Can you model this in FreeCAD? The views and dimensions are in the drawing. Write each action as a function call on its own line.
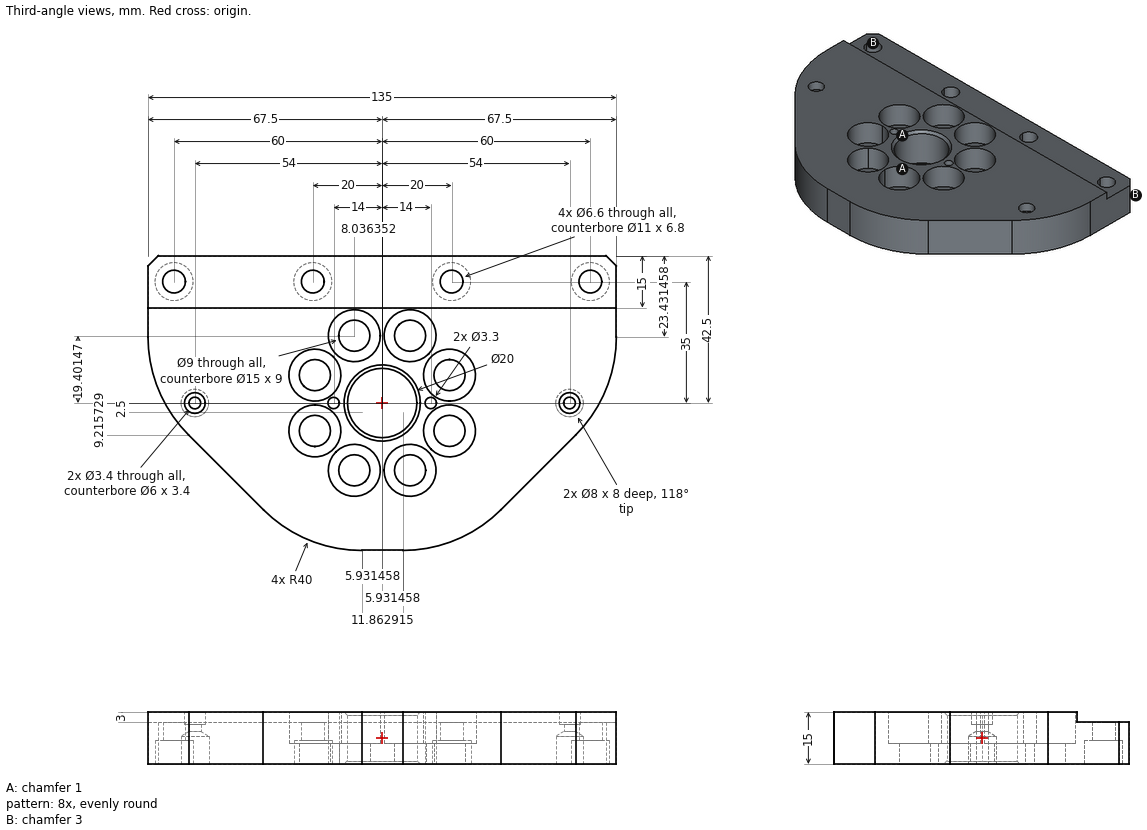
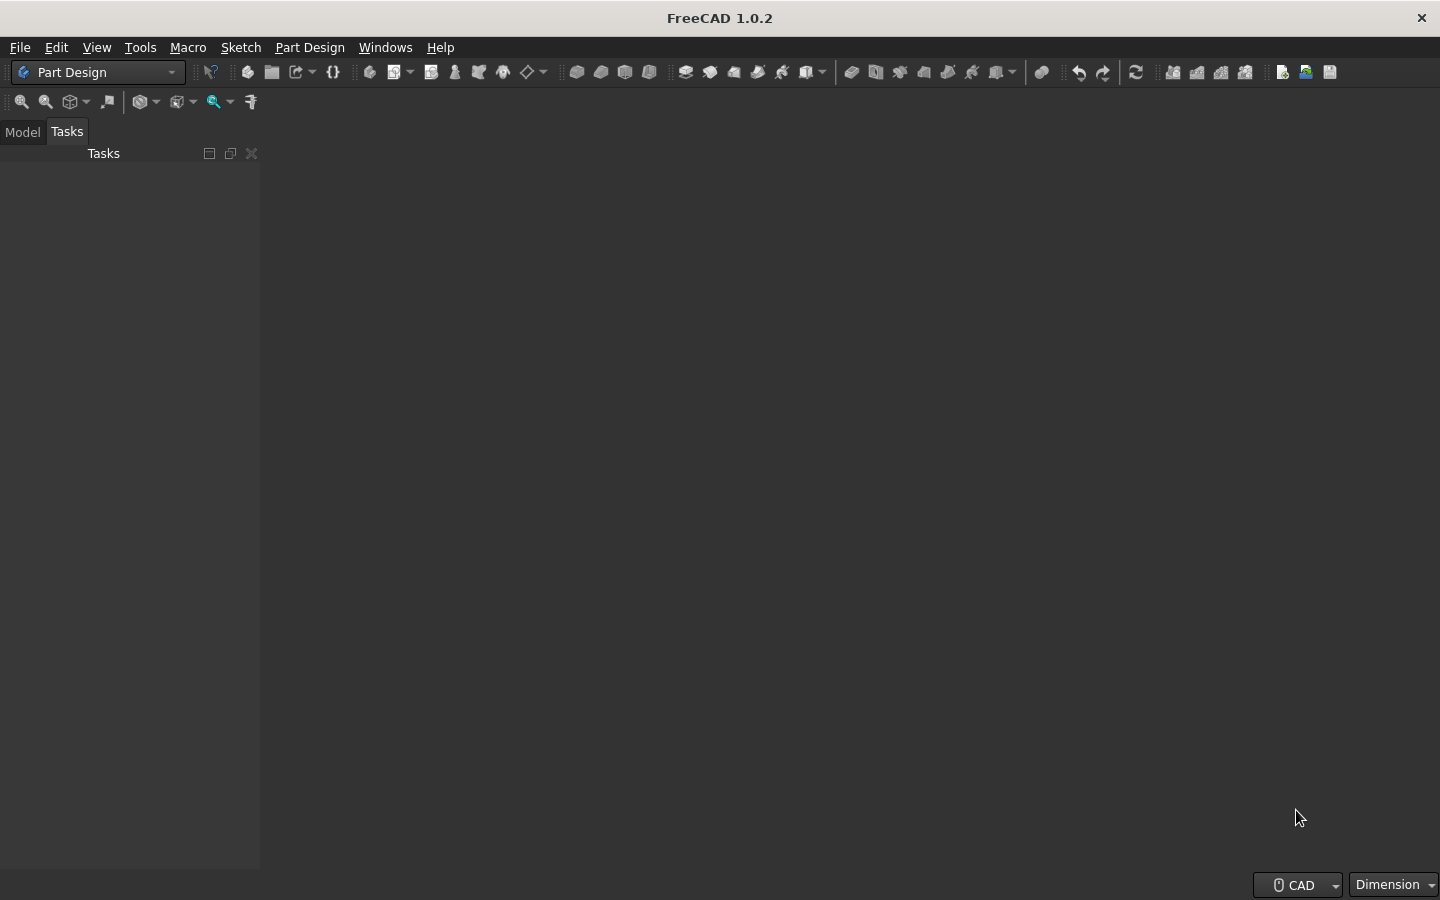
click(1282, 72)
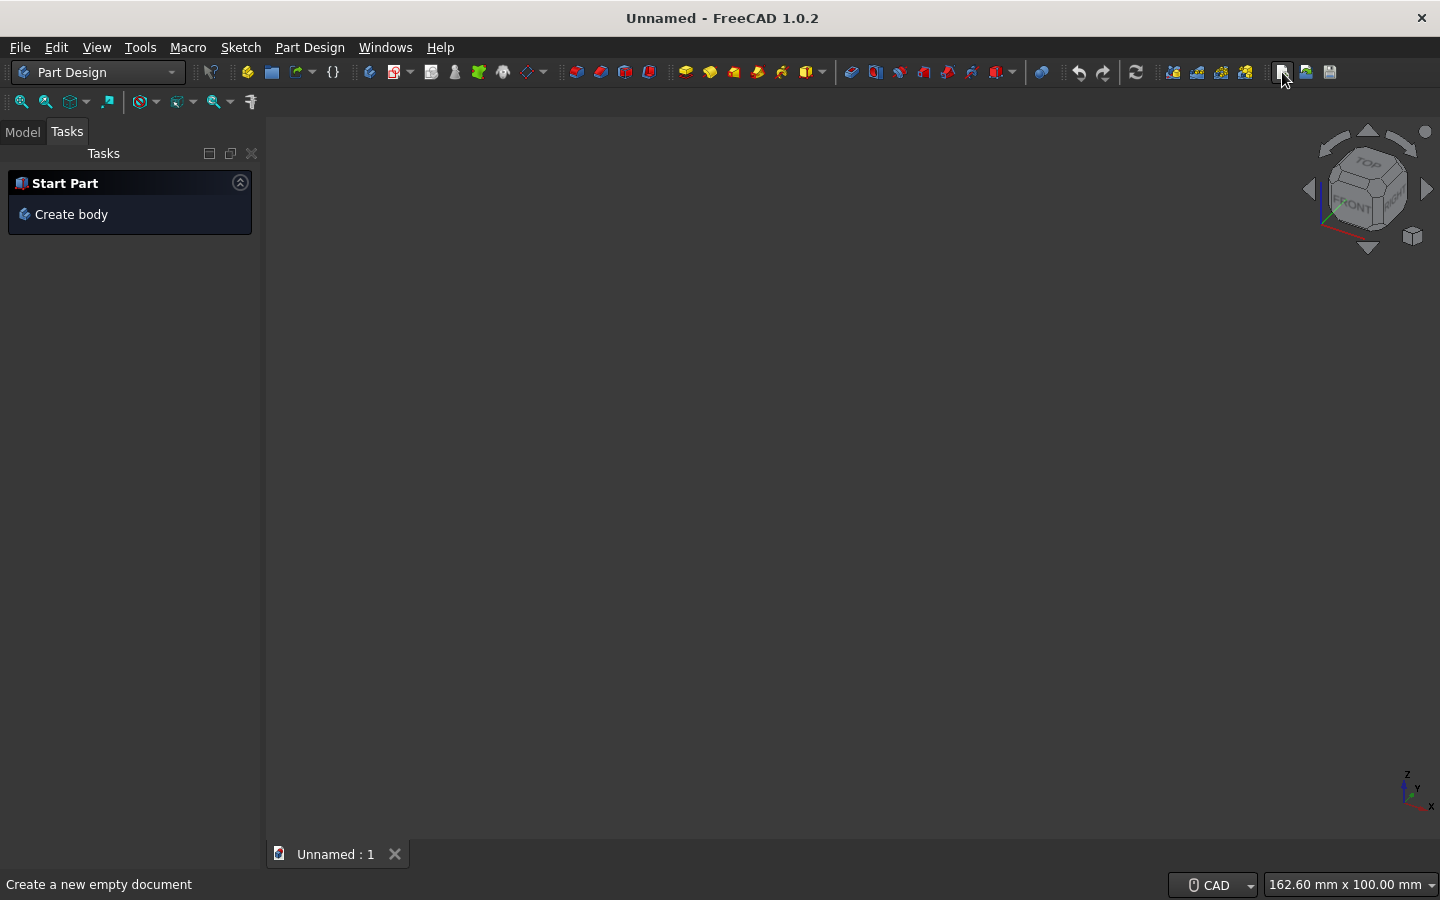
click(394, 72)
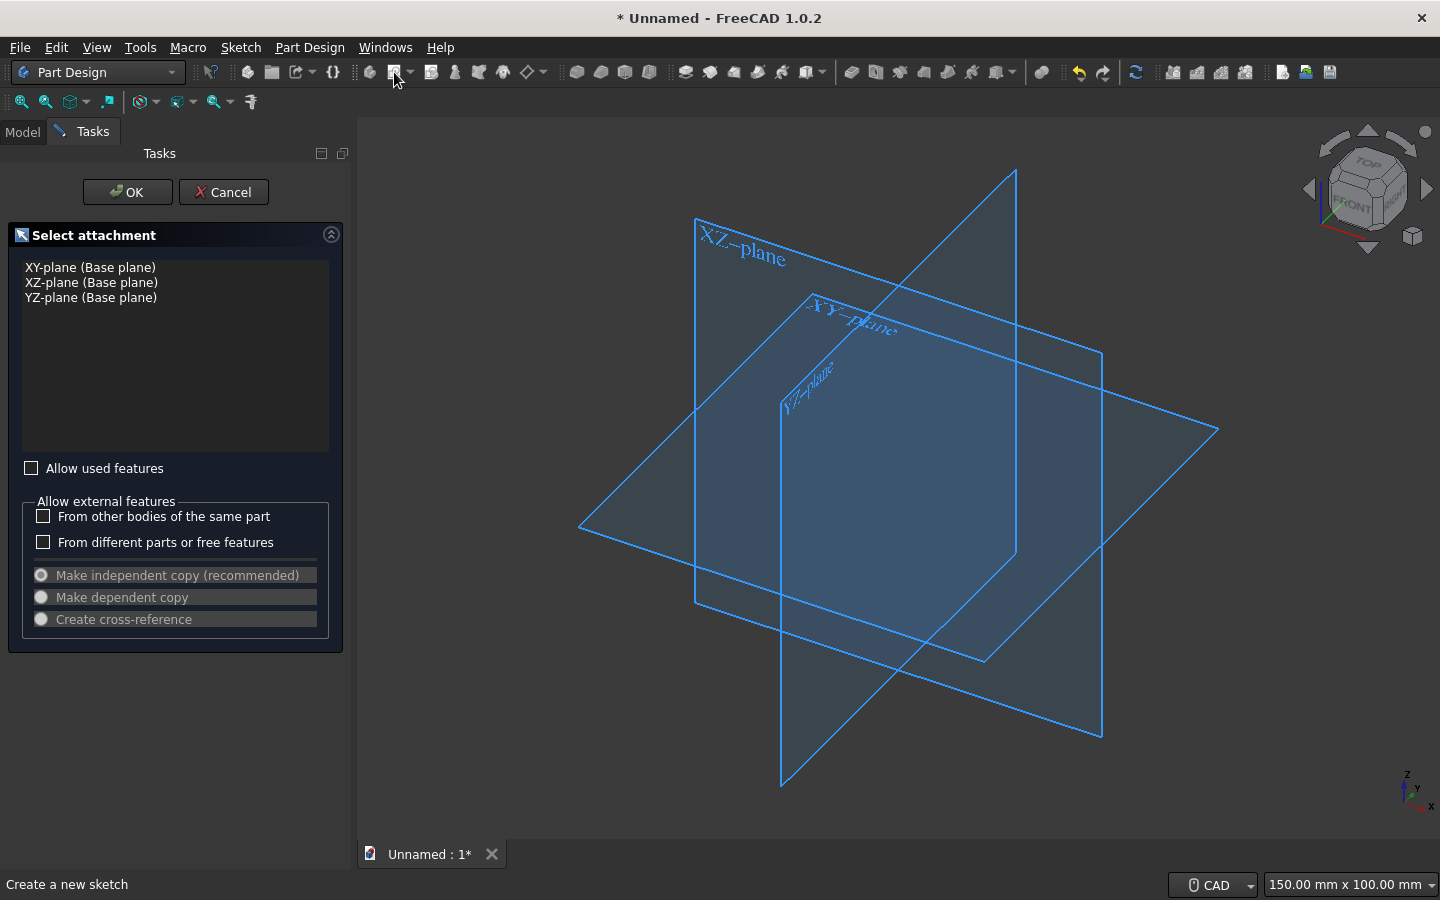
click(82, 268)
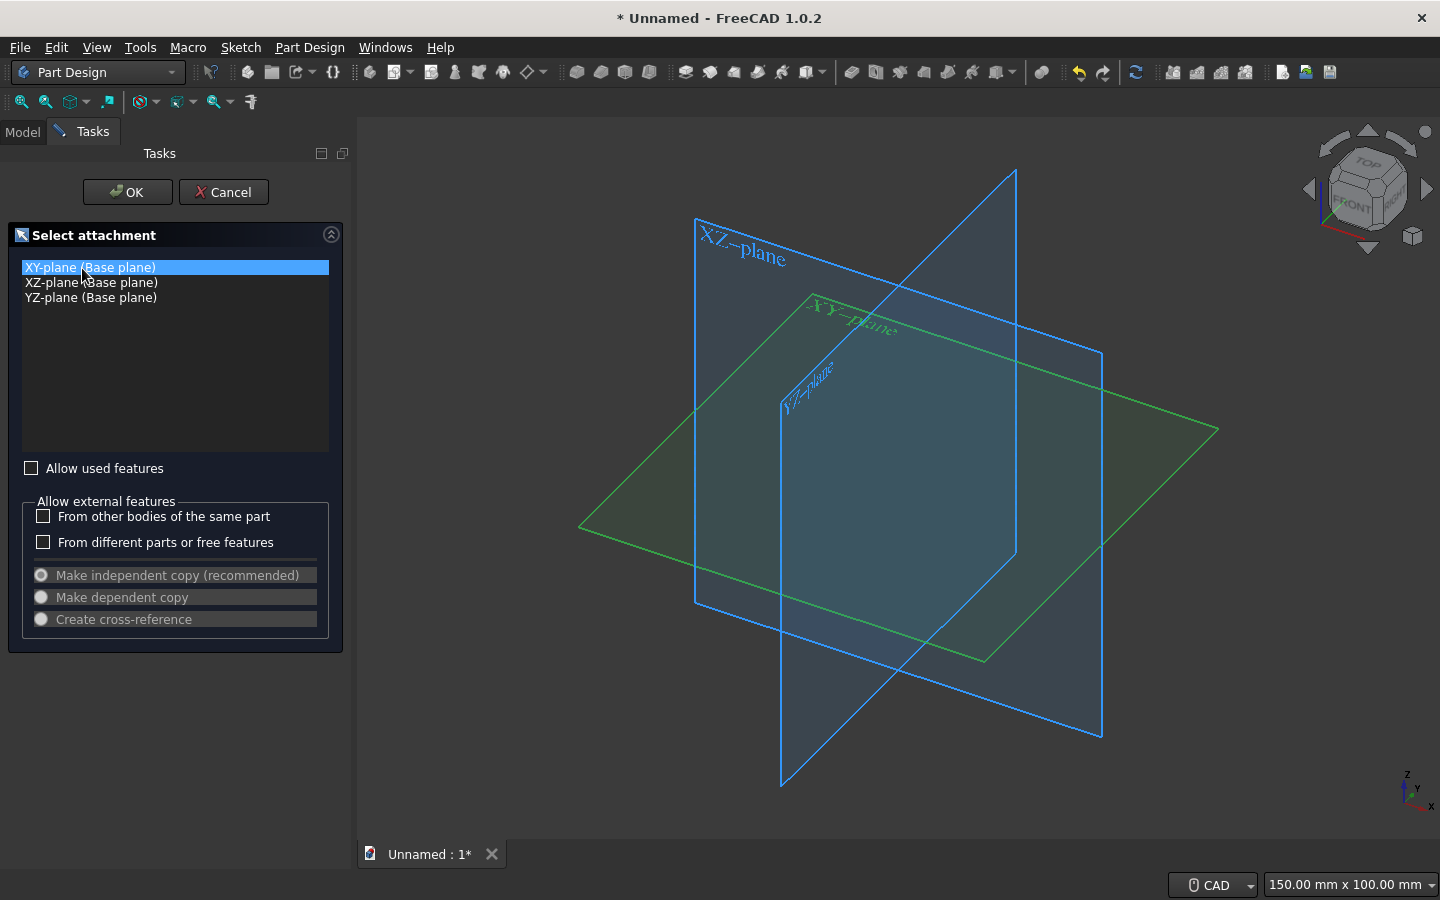
click(128, 192)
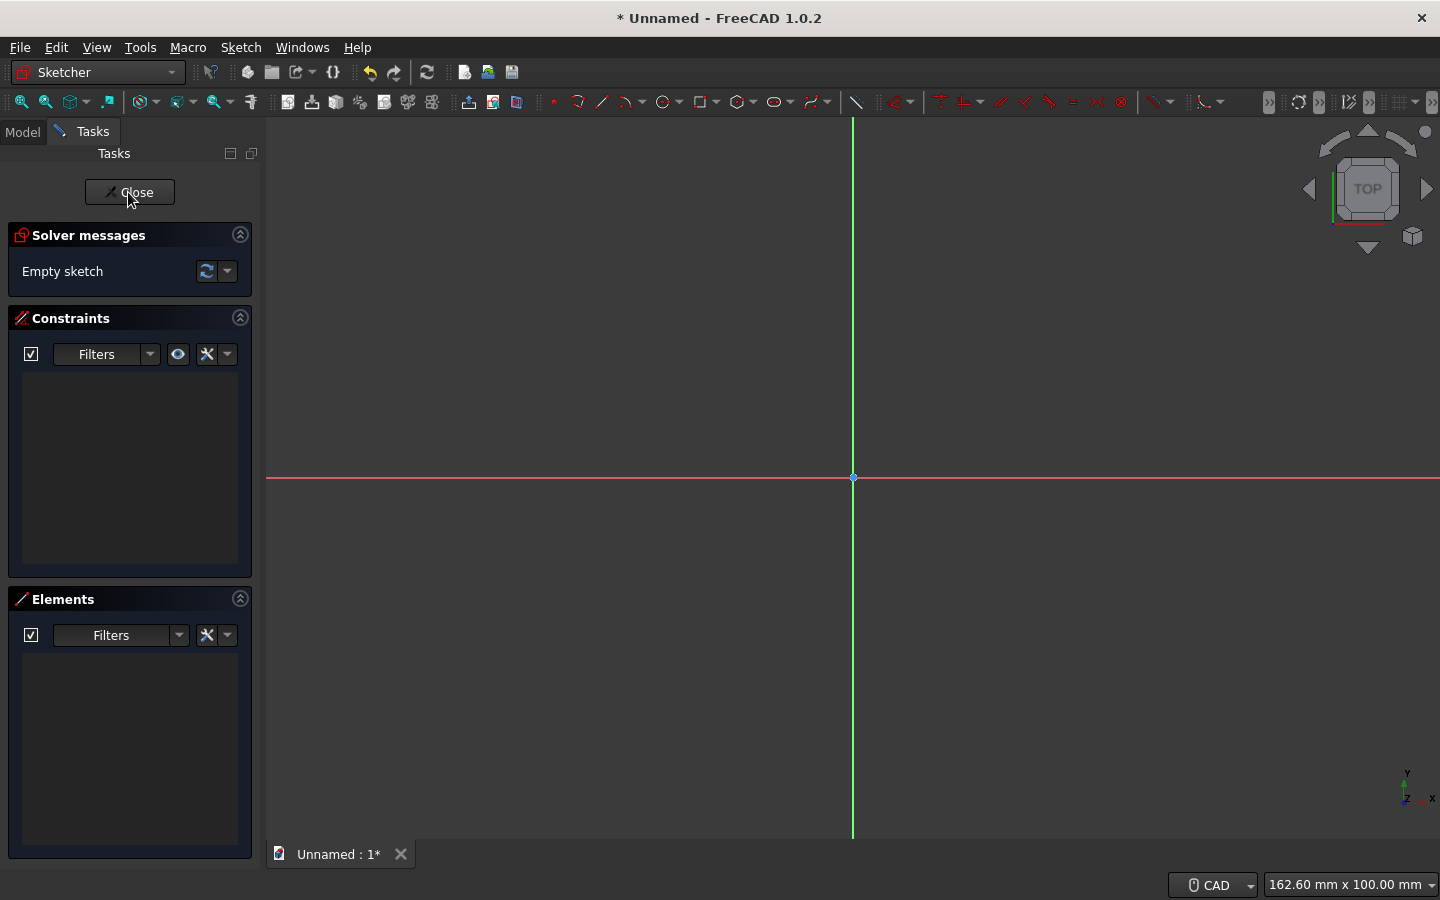
scroll(645, 478, down, 2)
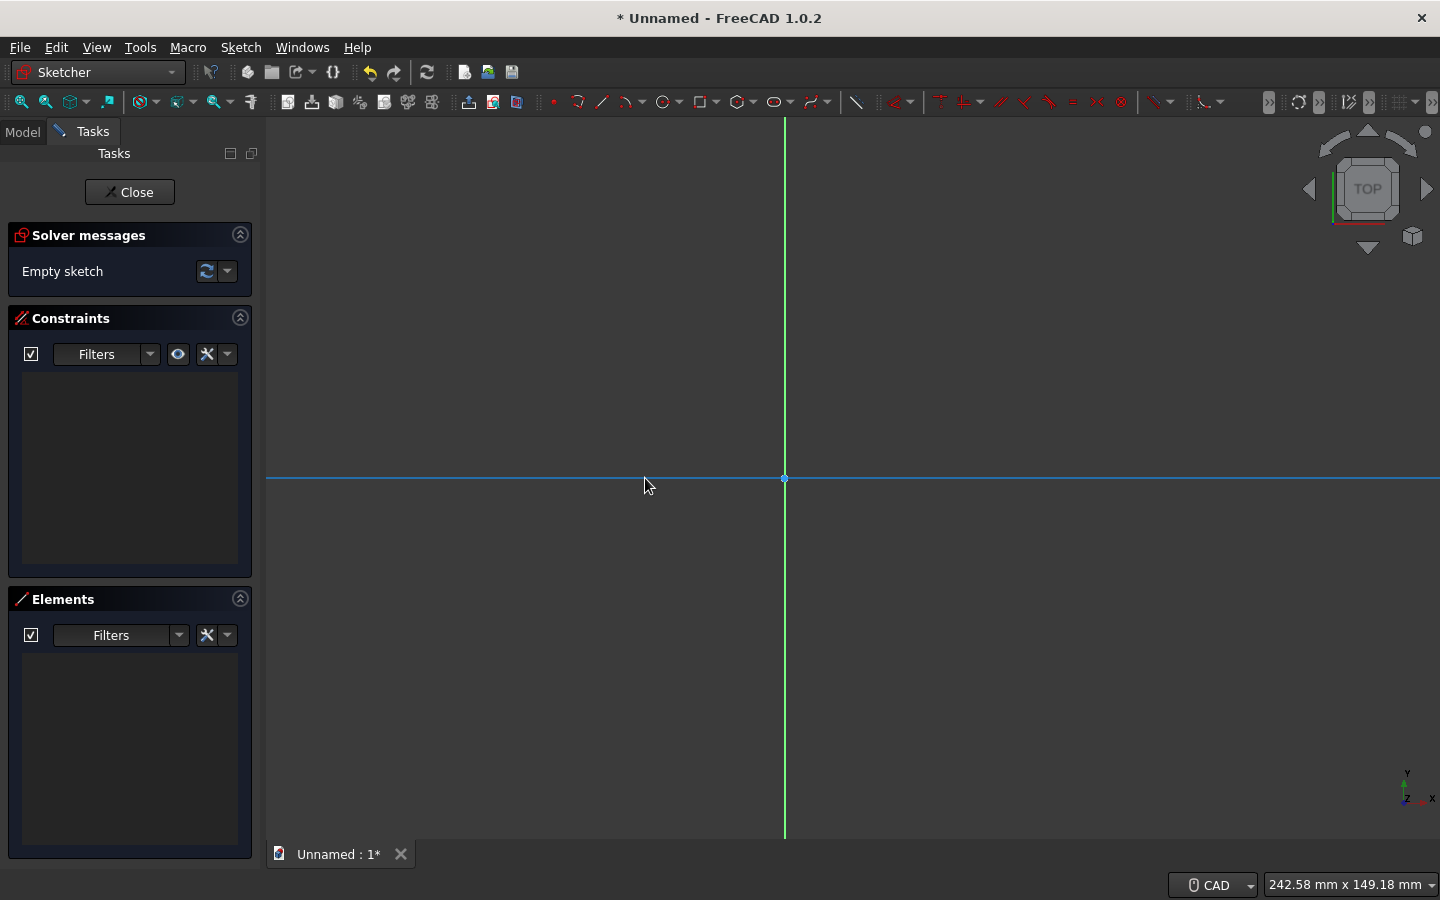
click(602, 102)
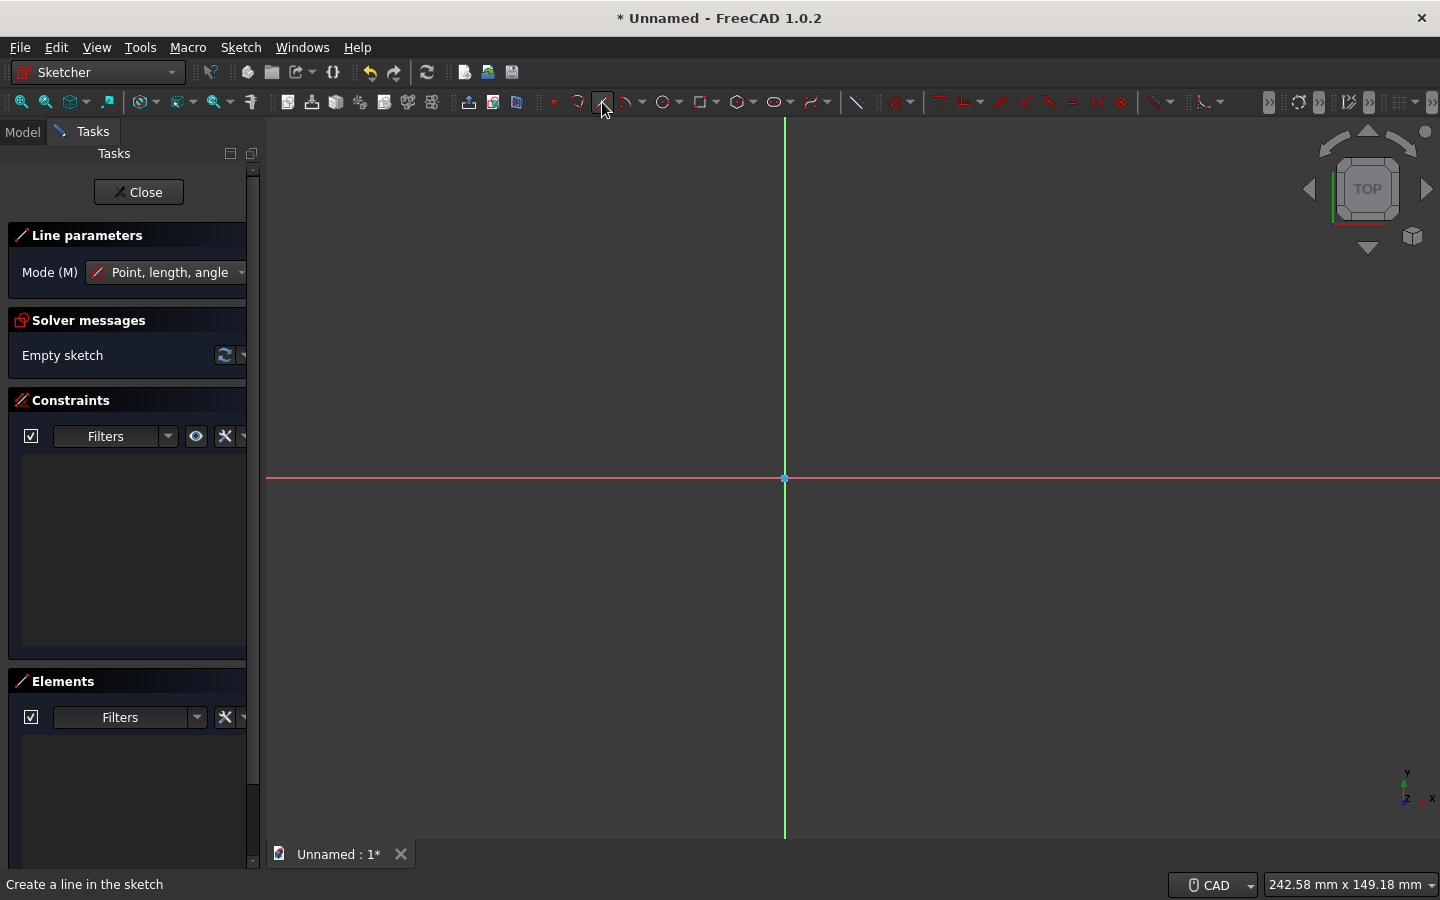
click(515, 523)
click(619, 627)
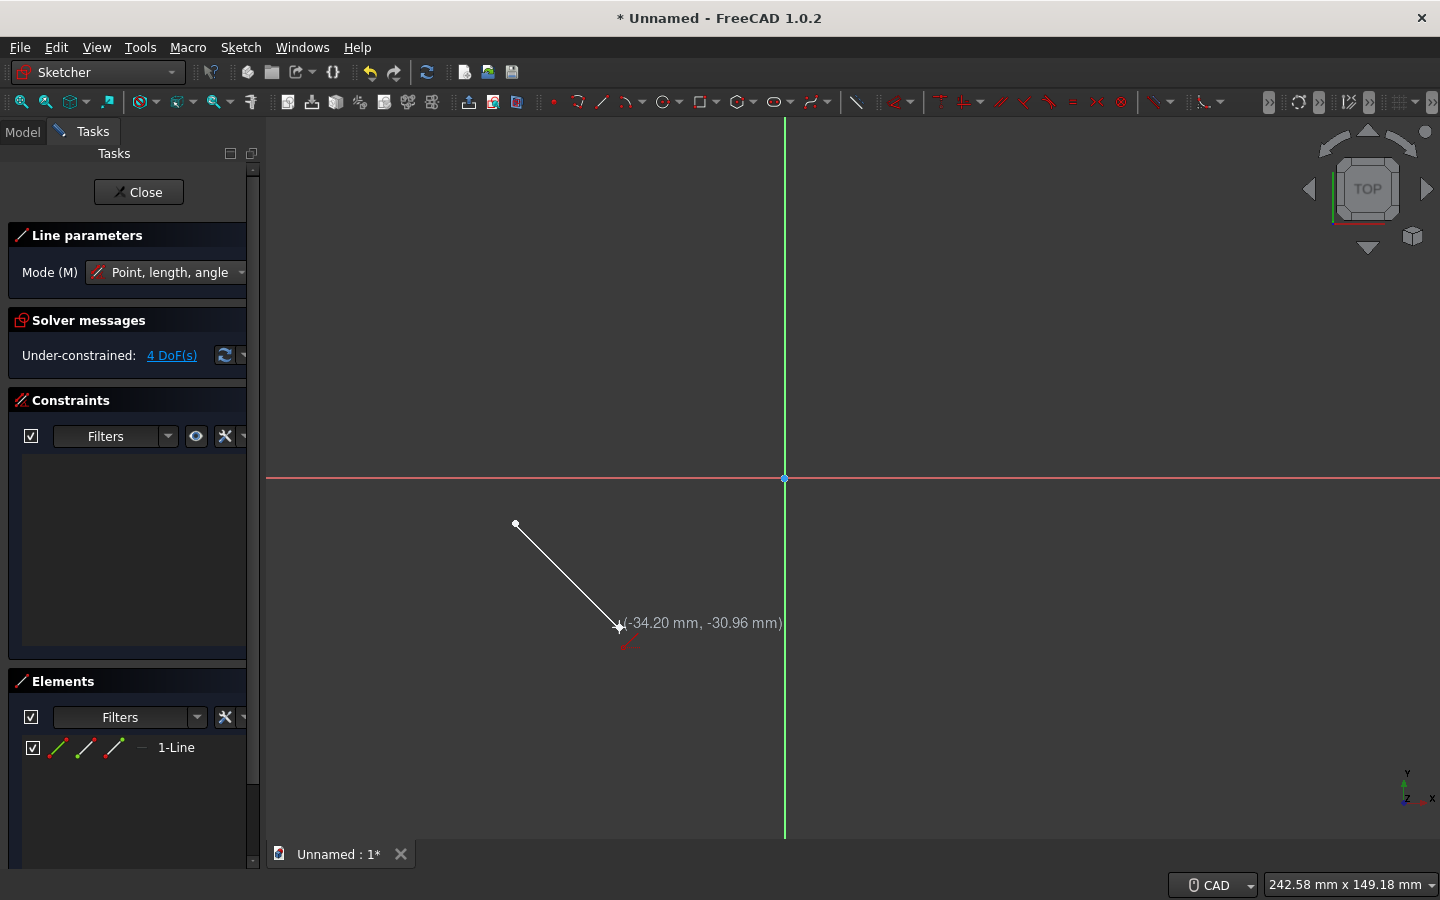
click(756, 684)
click(813, 684)